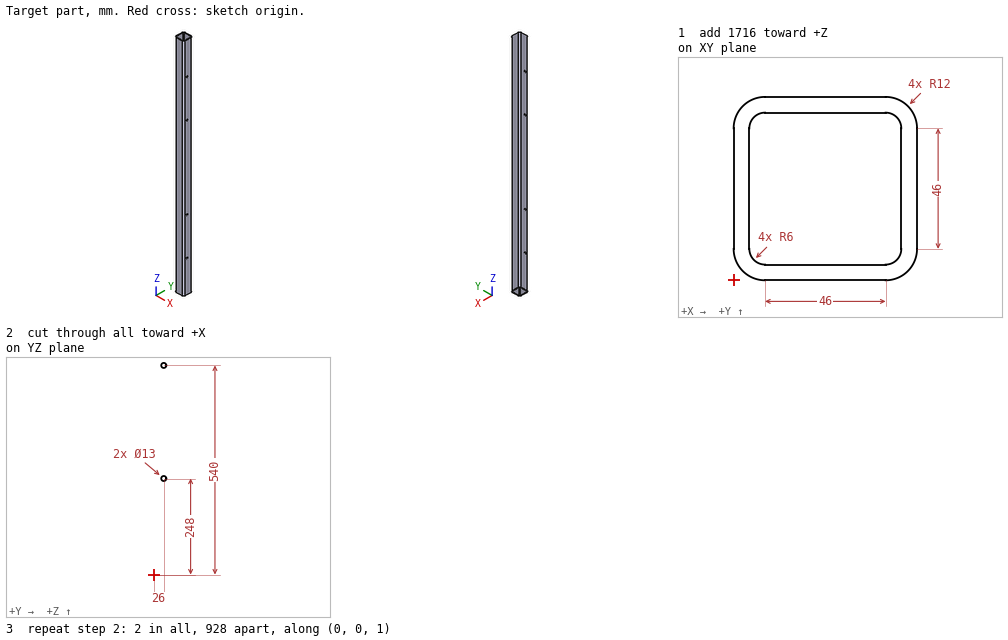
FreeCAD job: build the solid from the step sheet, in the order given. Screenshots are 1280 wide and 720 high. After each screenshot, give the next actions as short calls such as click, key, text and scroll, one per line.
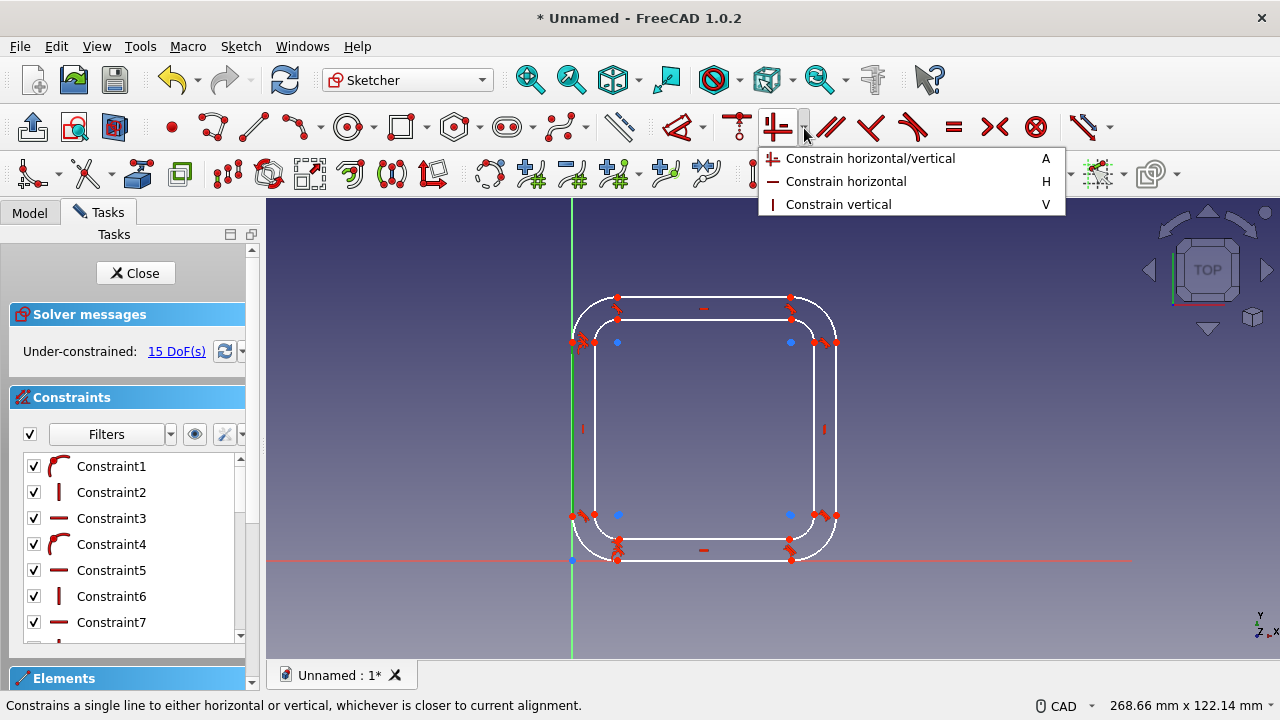
click(912, 204)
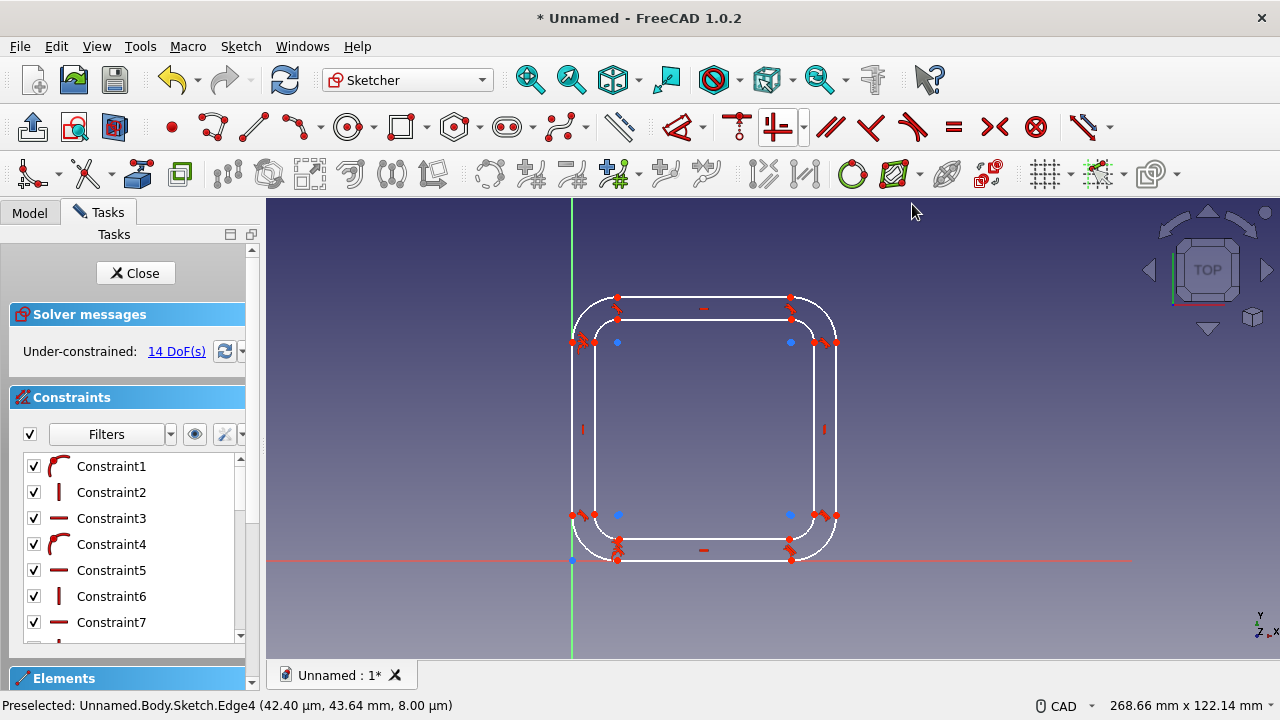
click(586, 548)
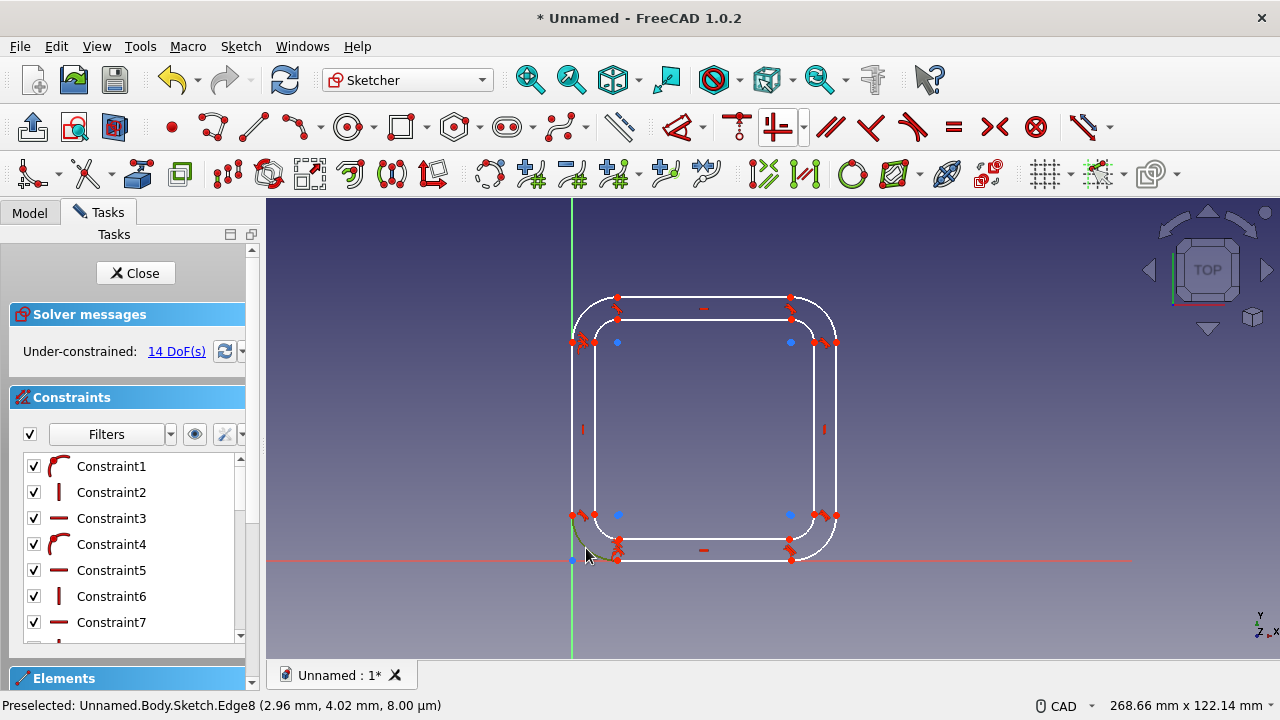
click(597, 526)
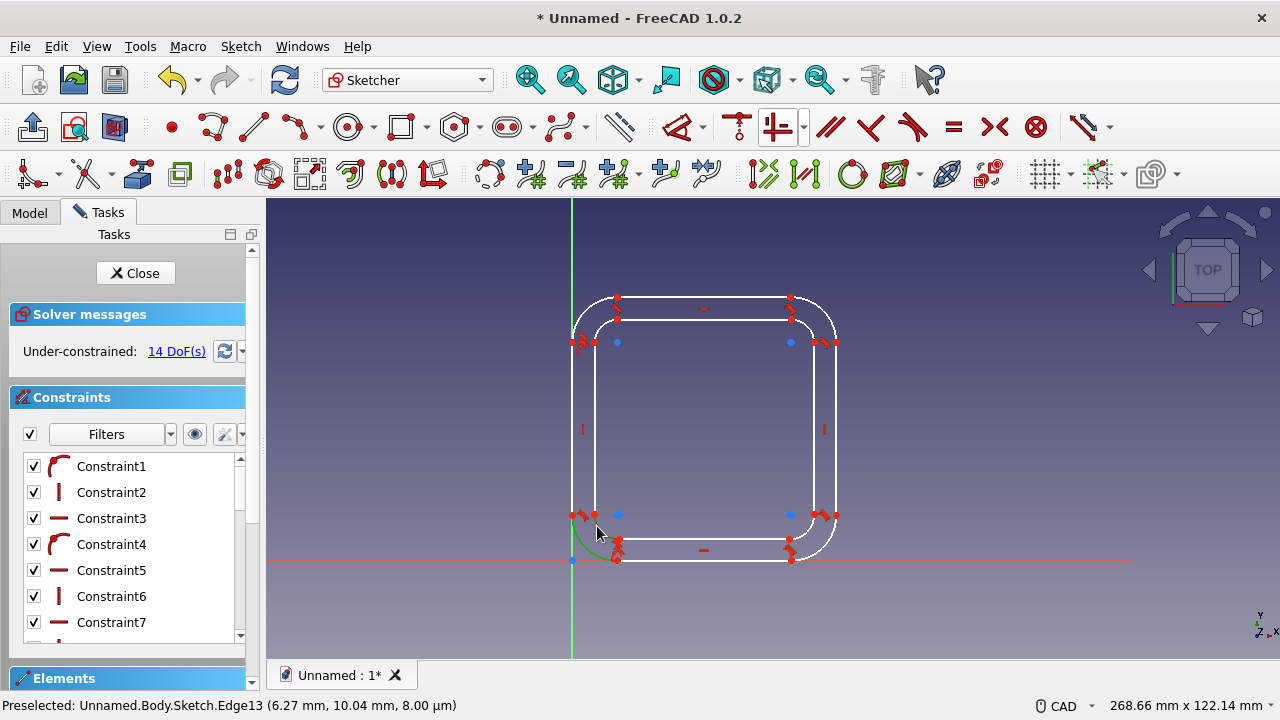
click(737, 128)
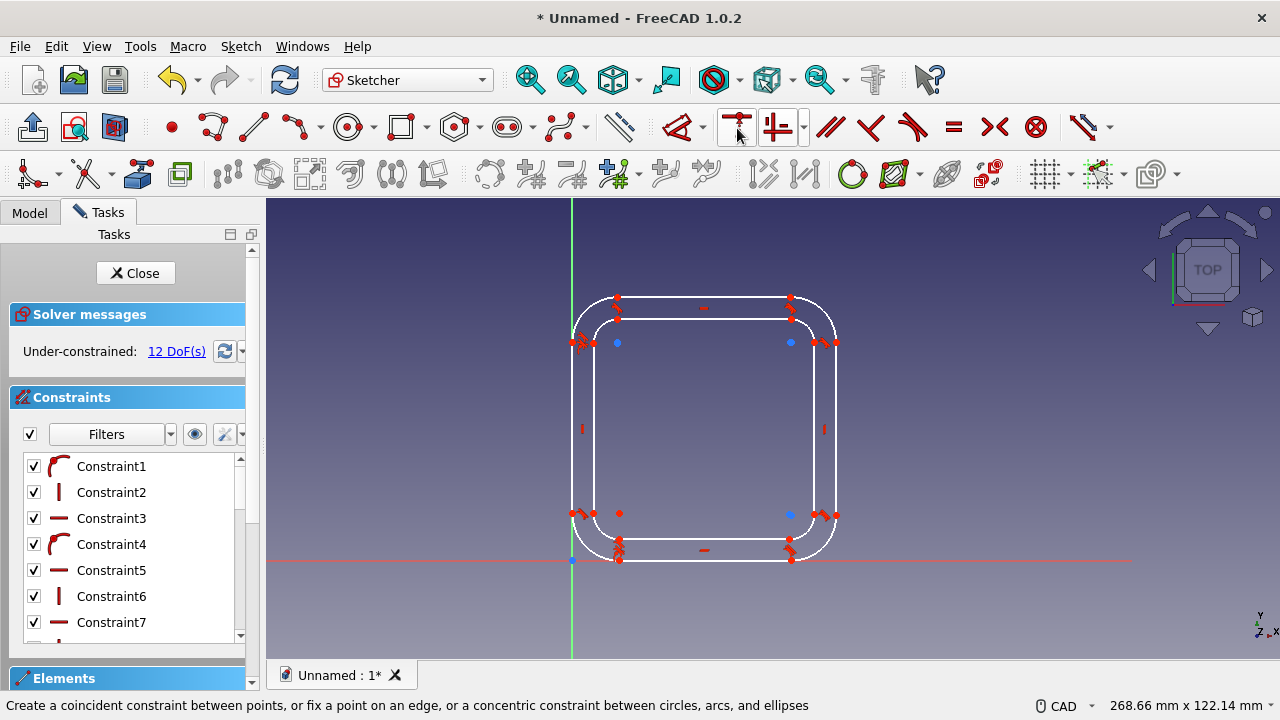
click(597, 302)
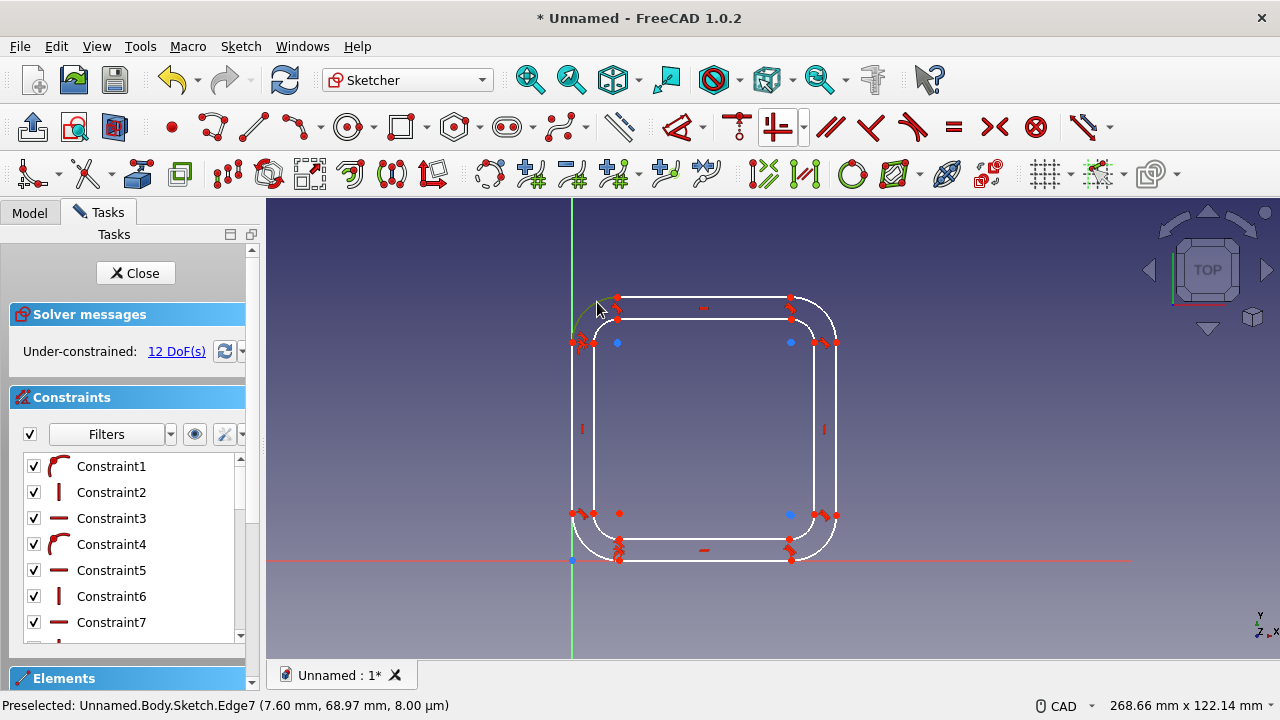
scroll(607, 322, up, 2)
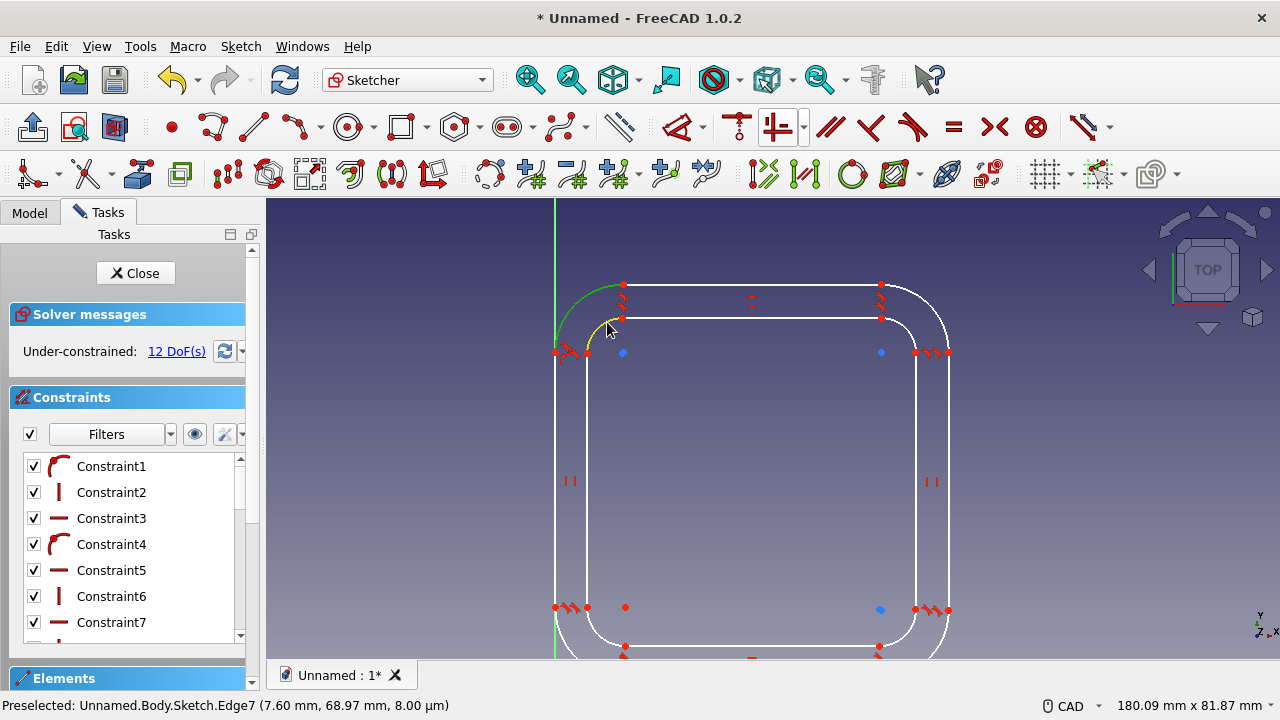
click(607, 322)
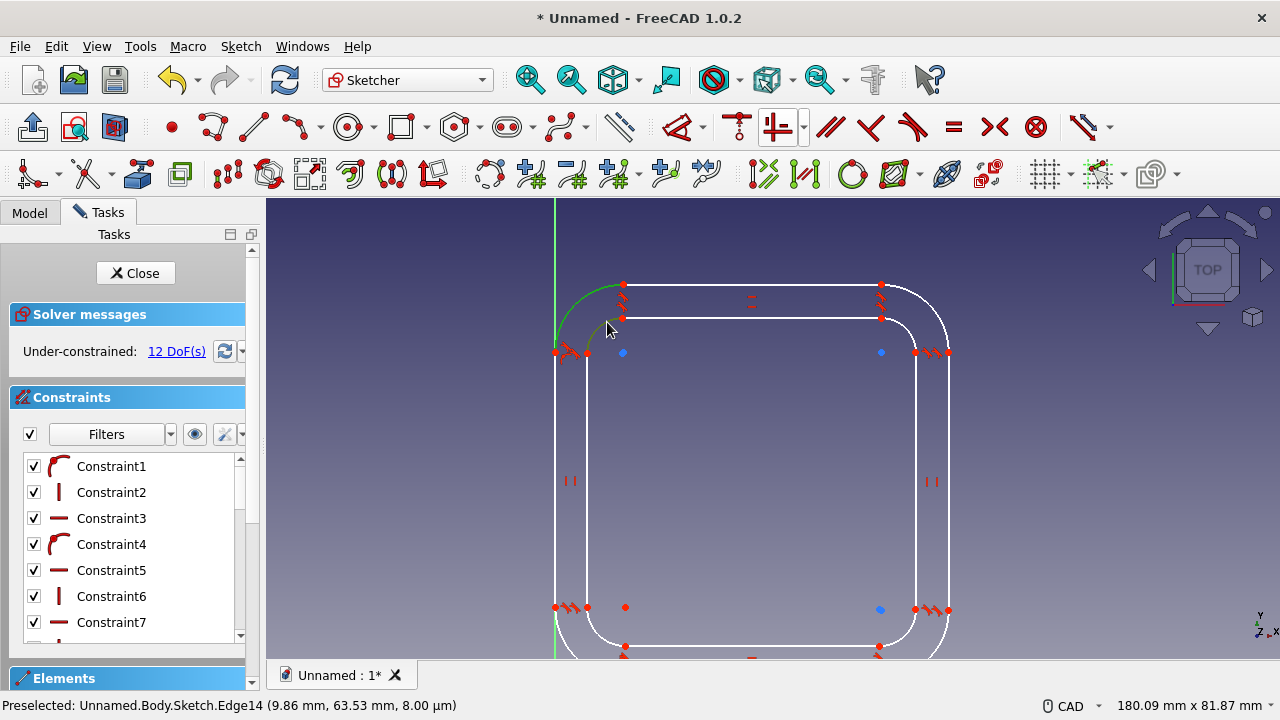
click(737, 128)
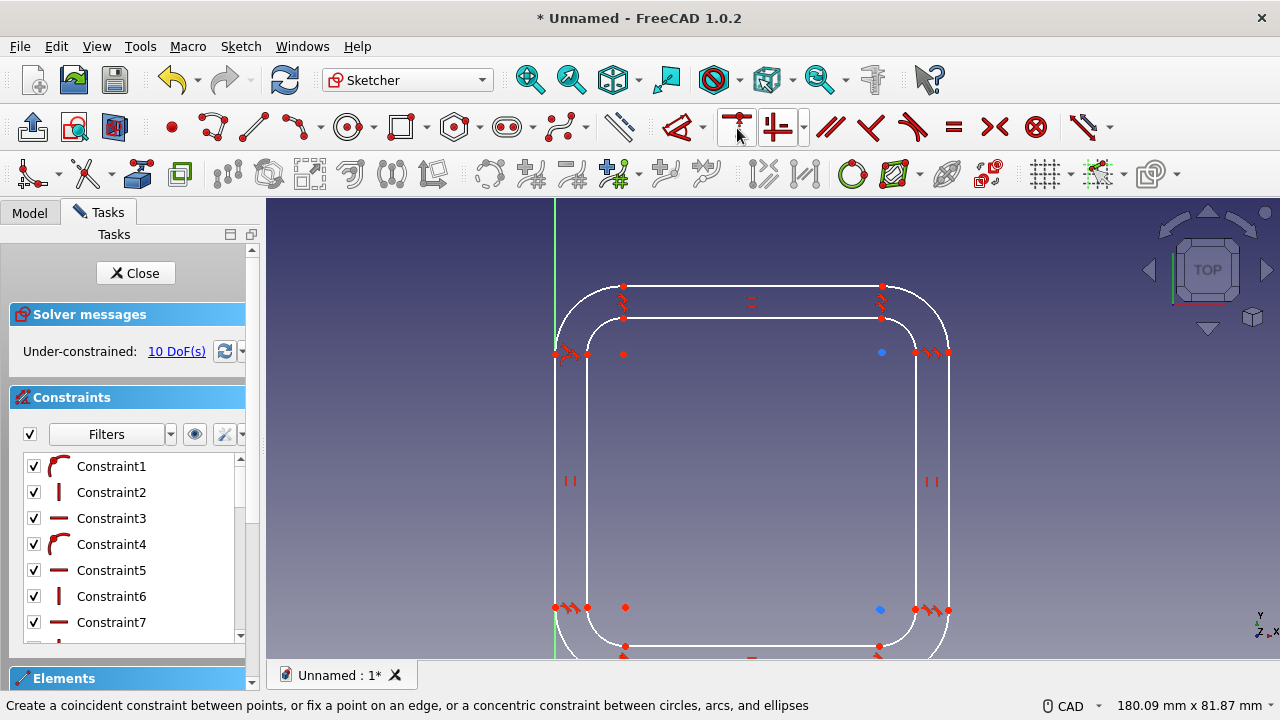
click(942, 322)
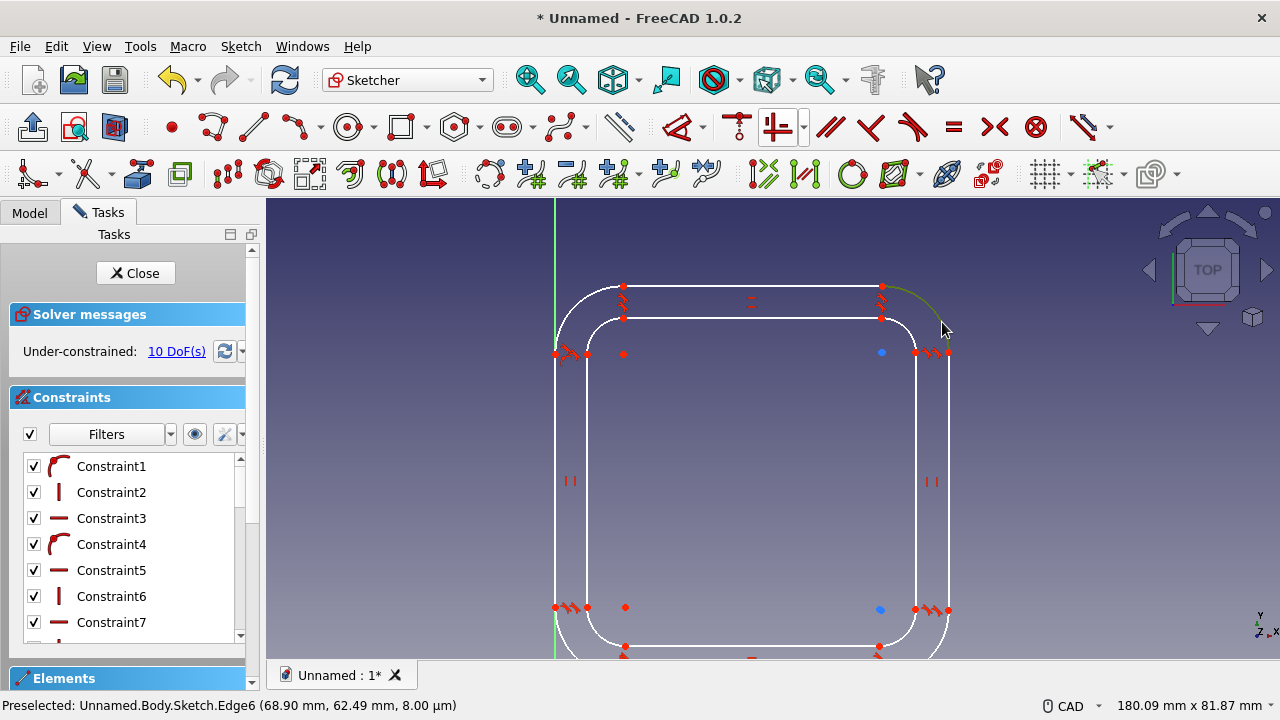
click(912, 337)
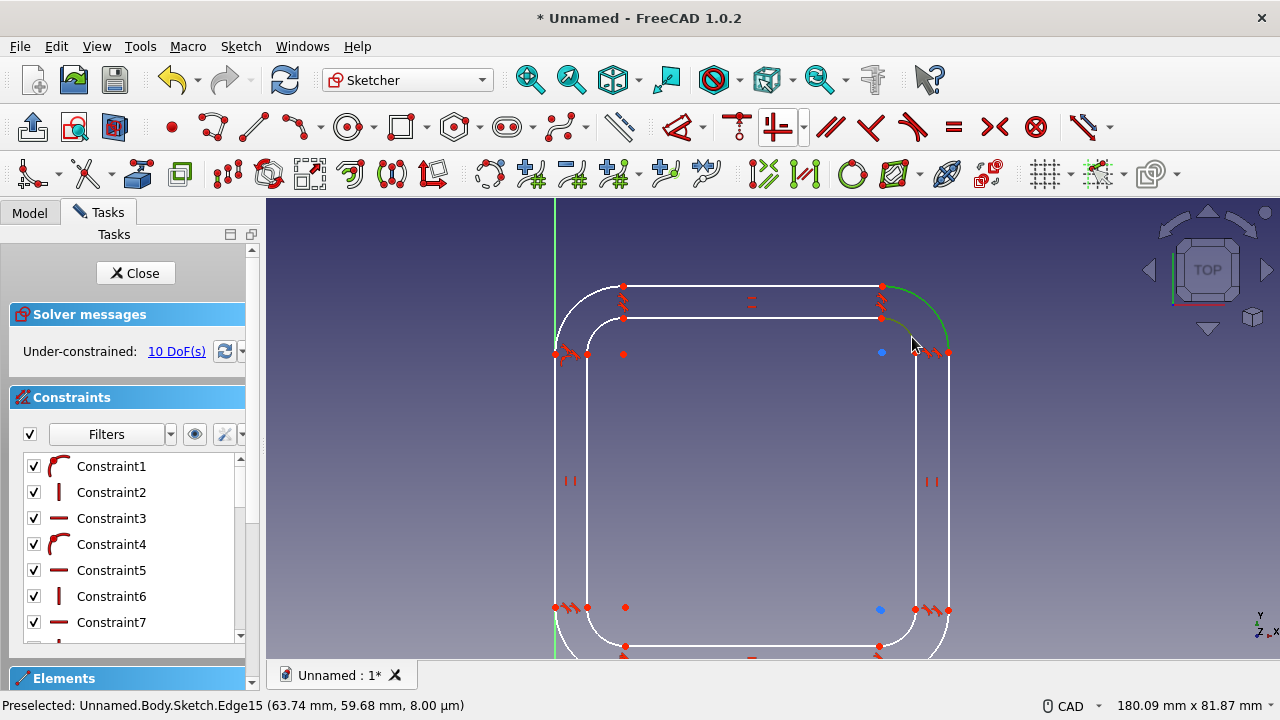
click(737, 128)